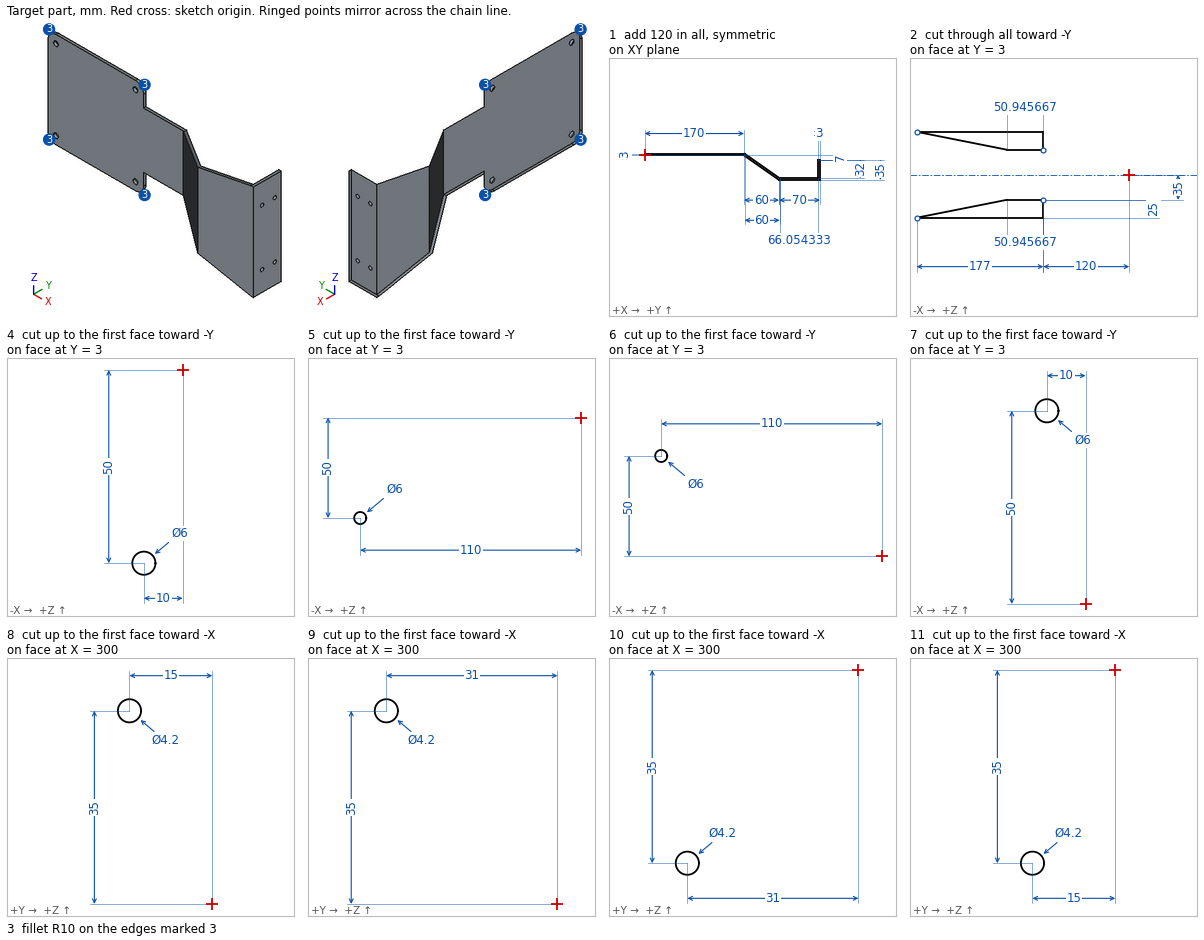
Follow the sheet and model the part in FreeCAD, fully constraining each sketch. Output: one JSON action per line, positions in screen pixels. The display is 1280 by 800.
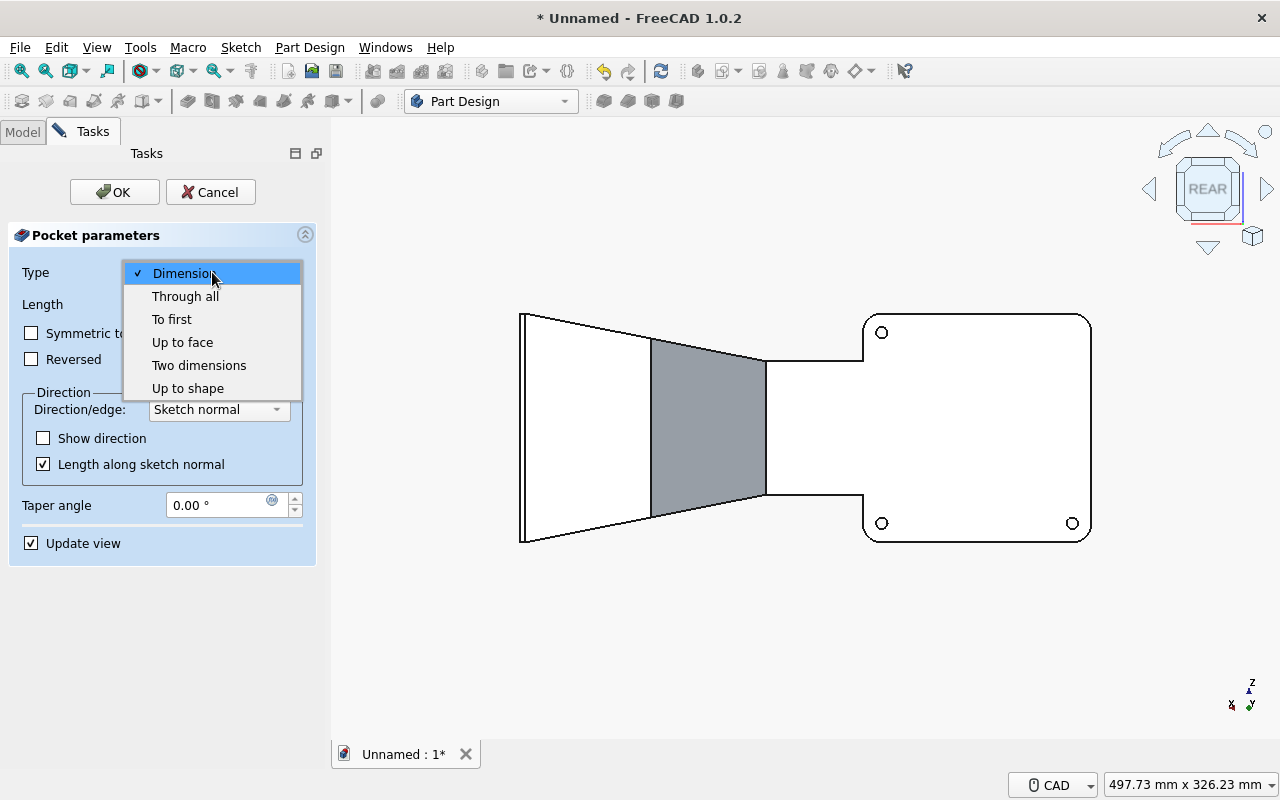
{"action": "left_click", "coordinate": [212, 320]}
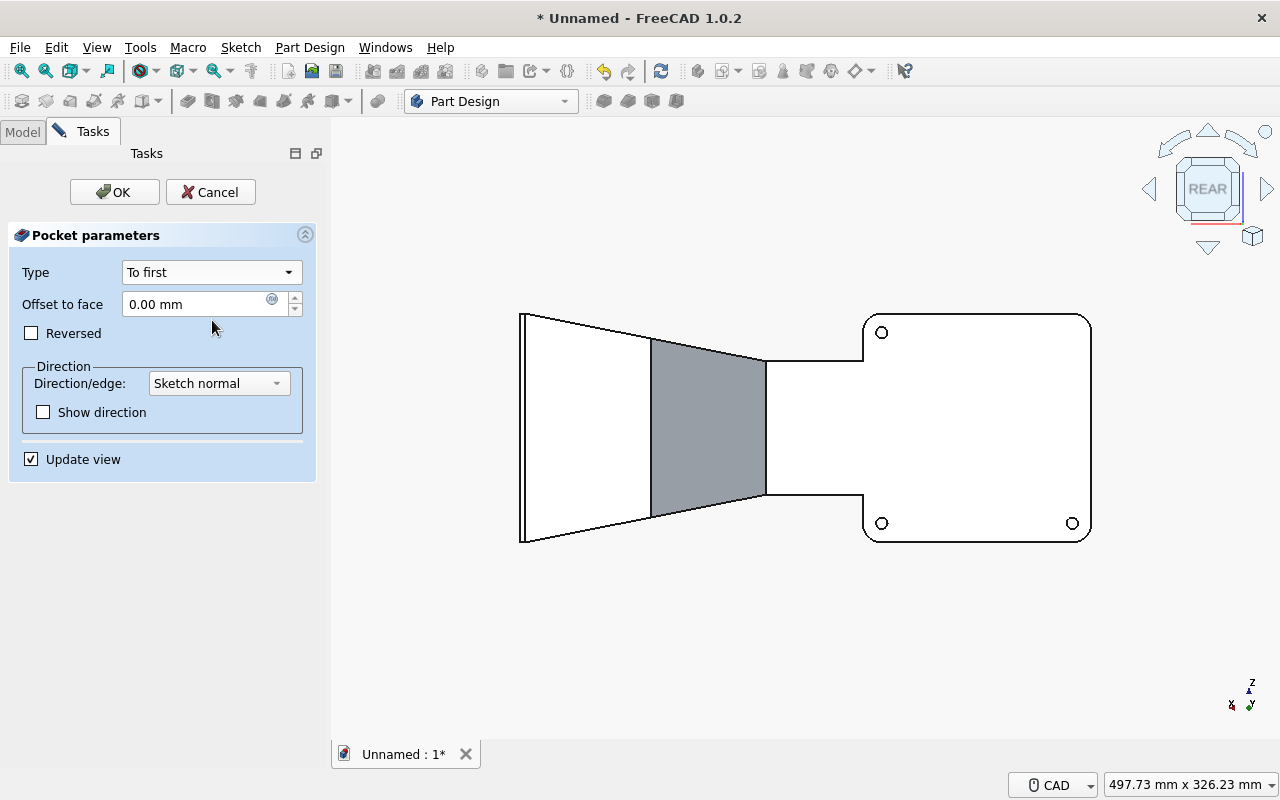
{"action": "left_click", "coordinate": [115, 192]}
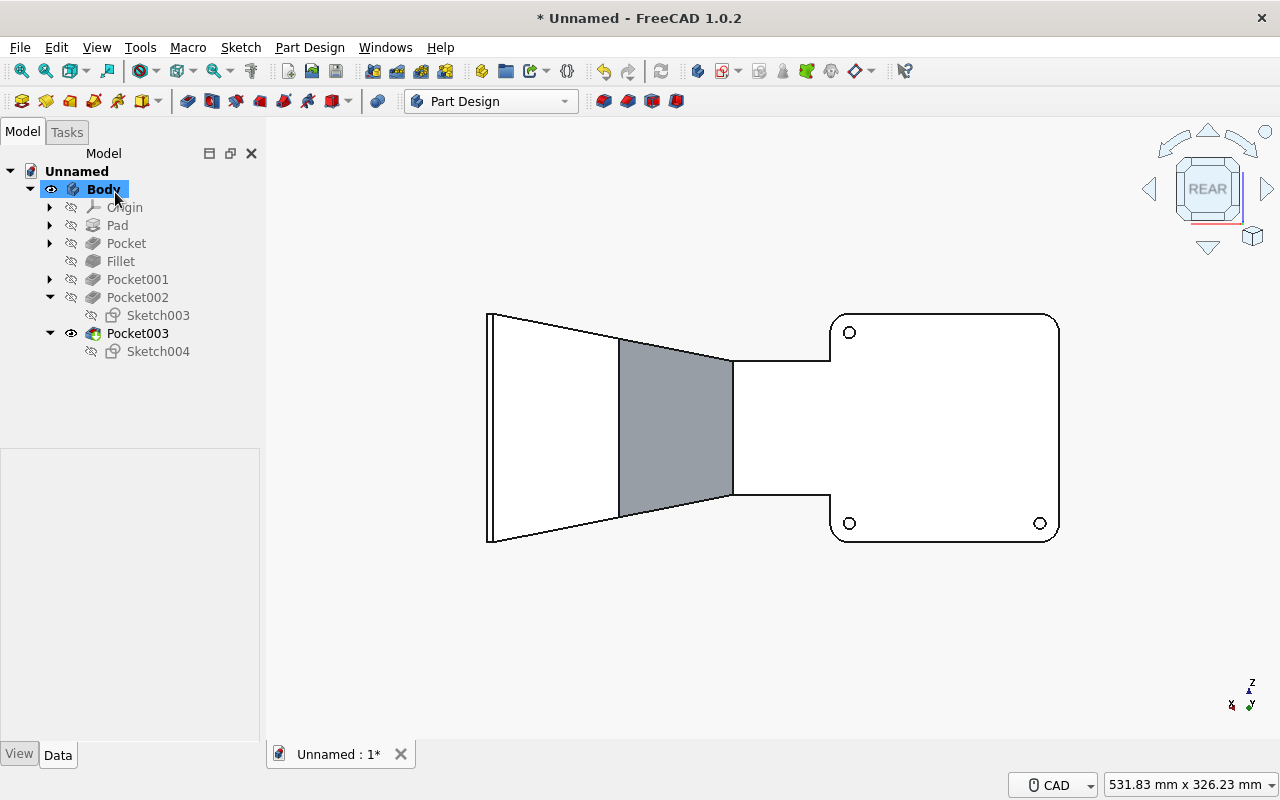
{"action": "left_click", "coordinate": [943, 427]}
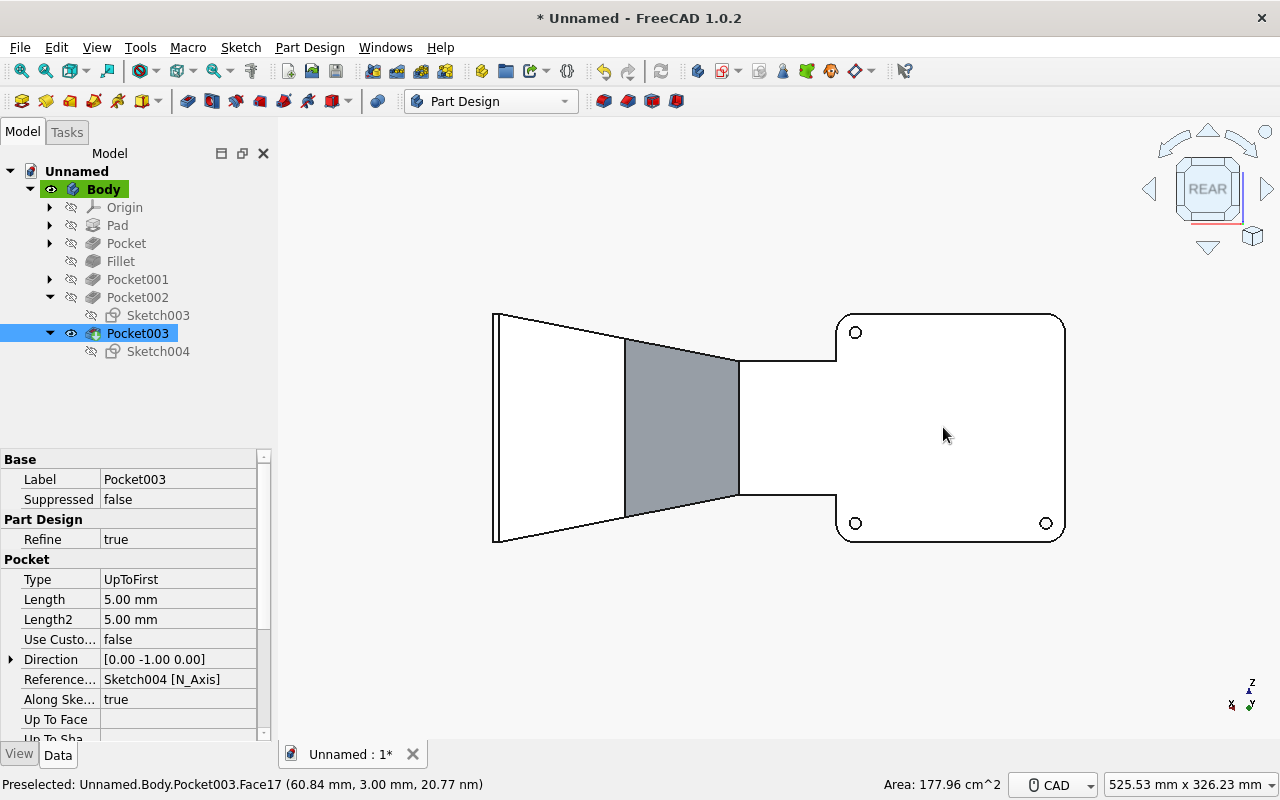
{"action": "left_click", "coordinate": [722, 72]}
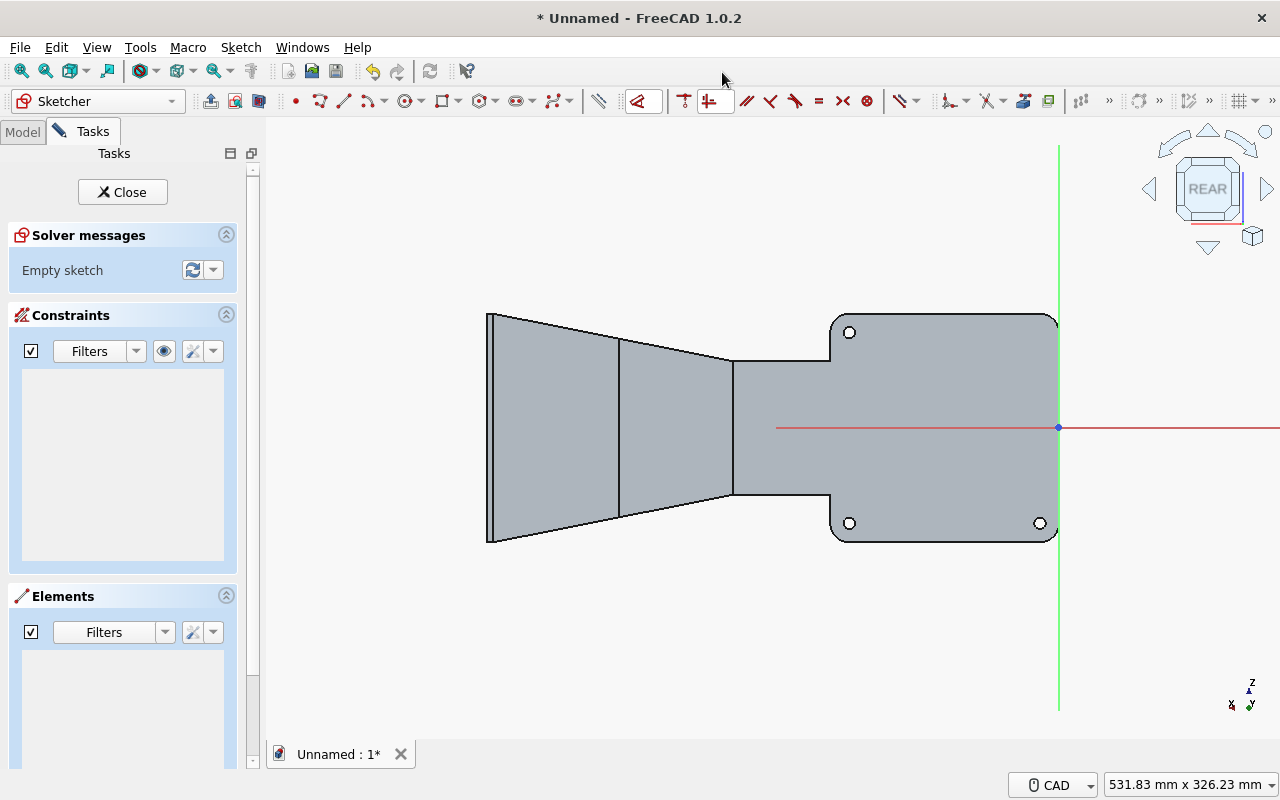
{"action": "scroll", "coordinate": [1058, 328], "scroll_direction": "up", "scroll_amount": 15}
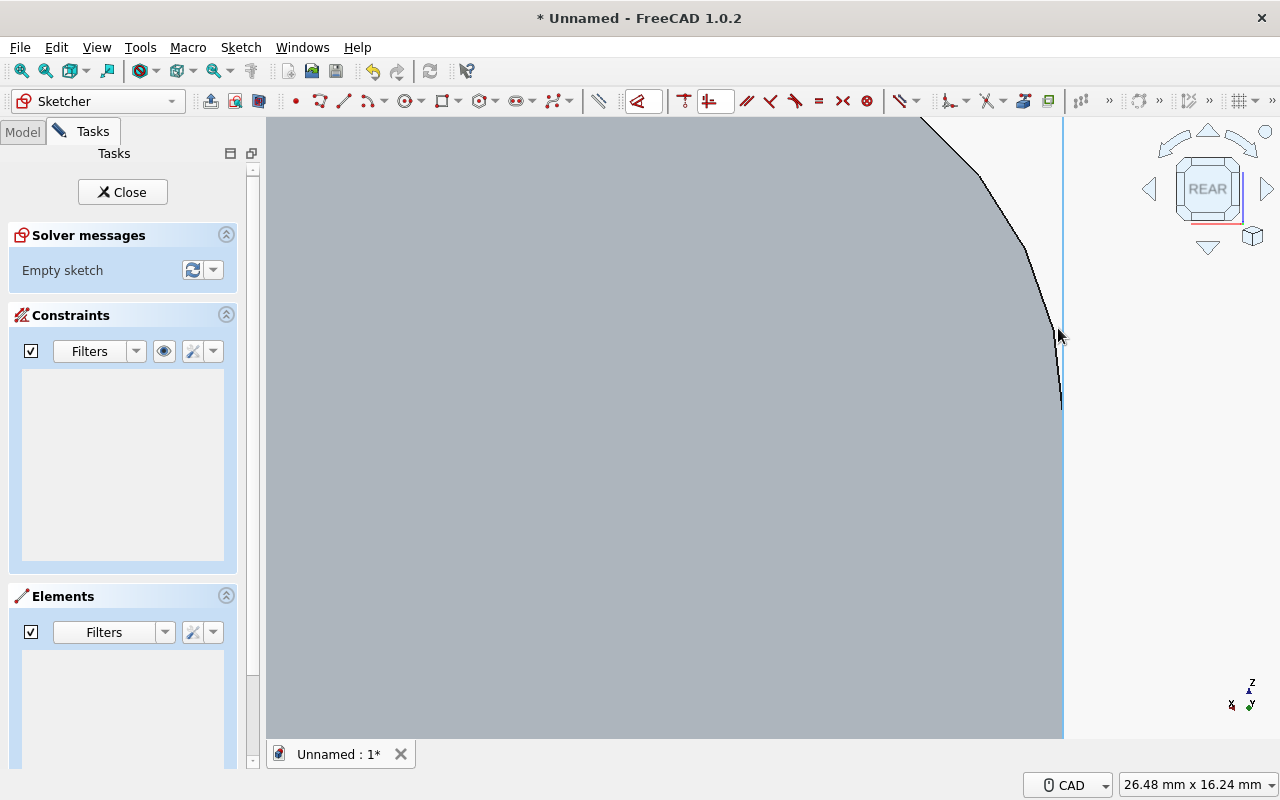
{"action": "scroll", "coordinate": [650, 400], "scroll_direction": "up", "scroll_amount": 3}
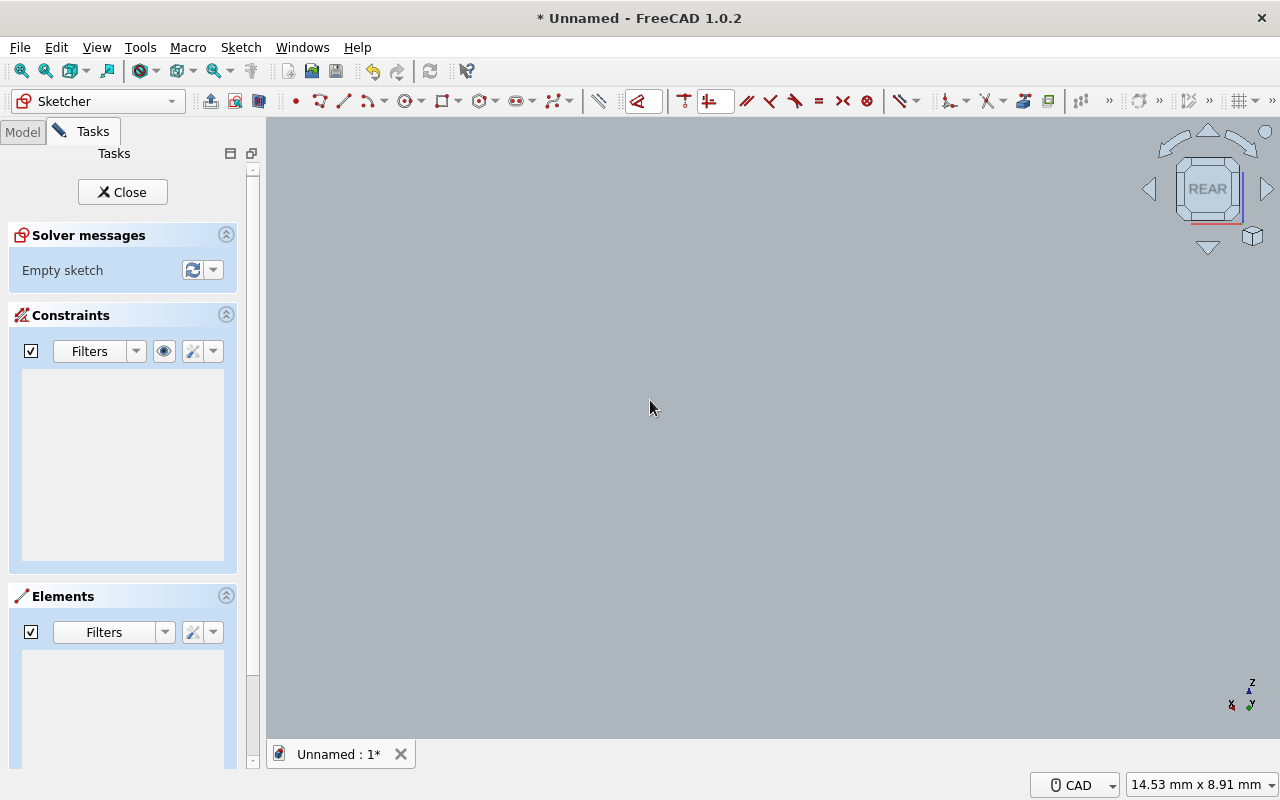
{"action": "left_click", "coordinate": [406, 102]}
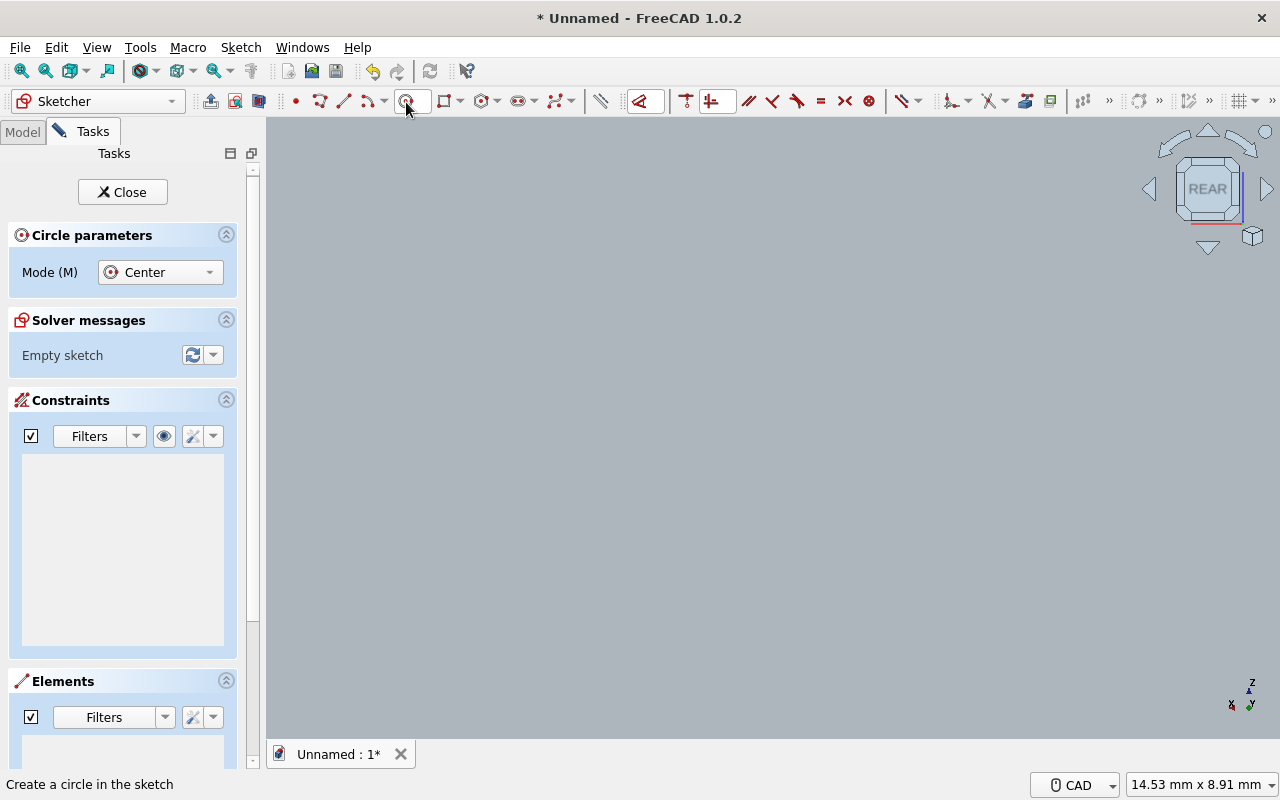
{"action": "left_click", "coordinate": [705, 427]}
{"action": "left_click", "coordinate": [853, 279]}
{"action": "key", "text": "Escape"}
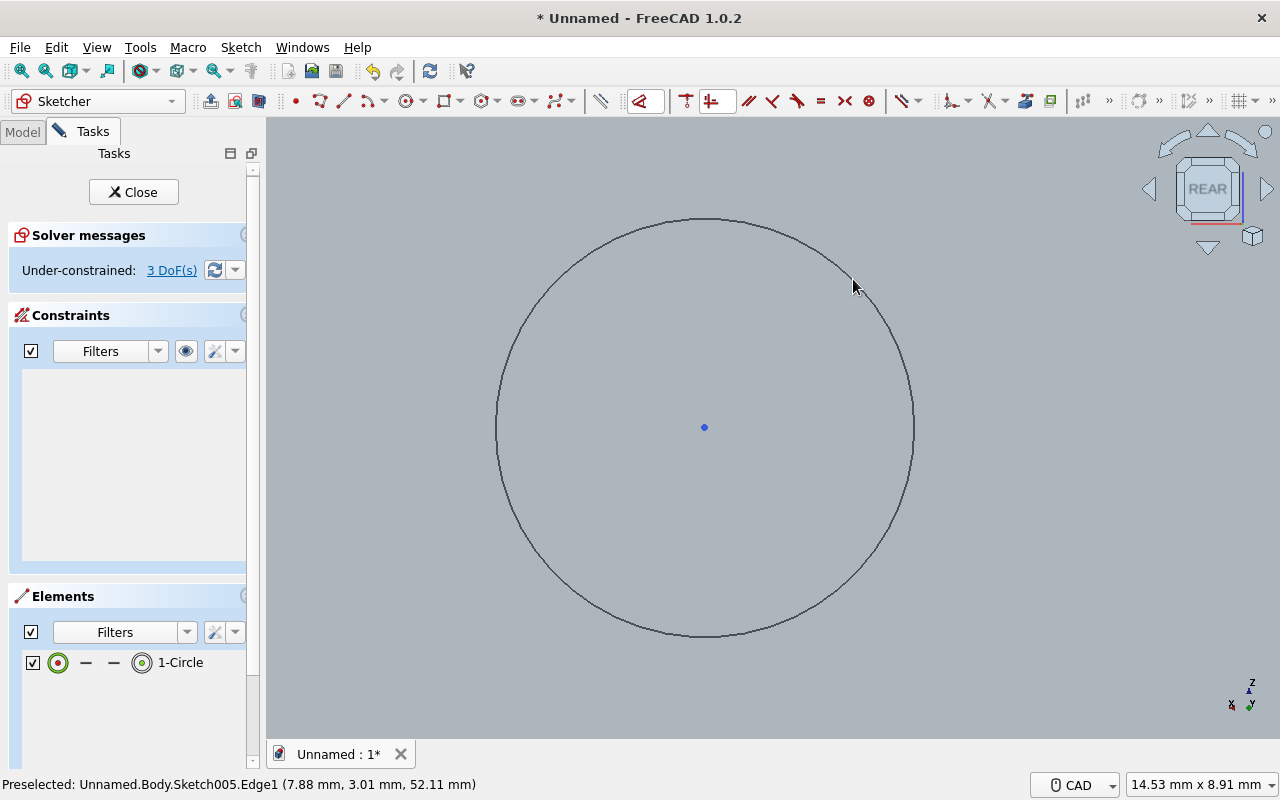
{"action": "left_click", "coordinate": [853, 280]}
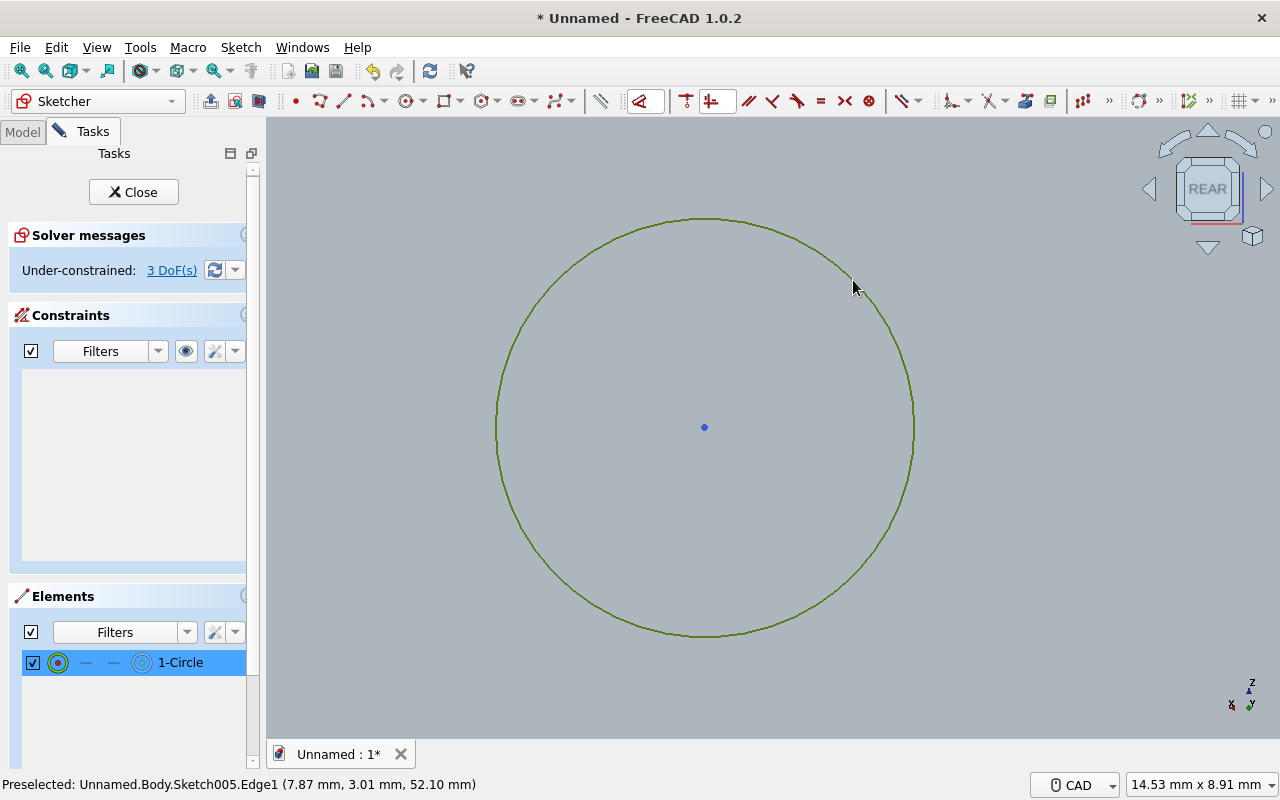
{"action": "left_click", "coordinate": [658, 102]}